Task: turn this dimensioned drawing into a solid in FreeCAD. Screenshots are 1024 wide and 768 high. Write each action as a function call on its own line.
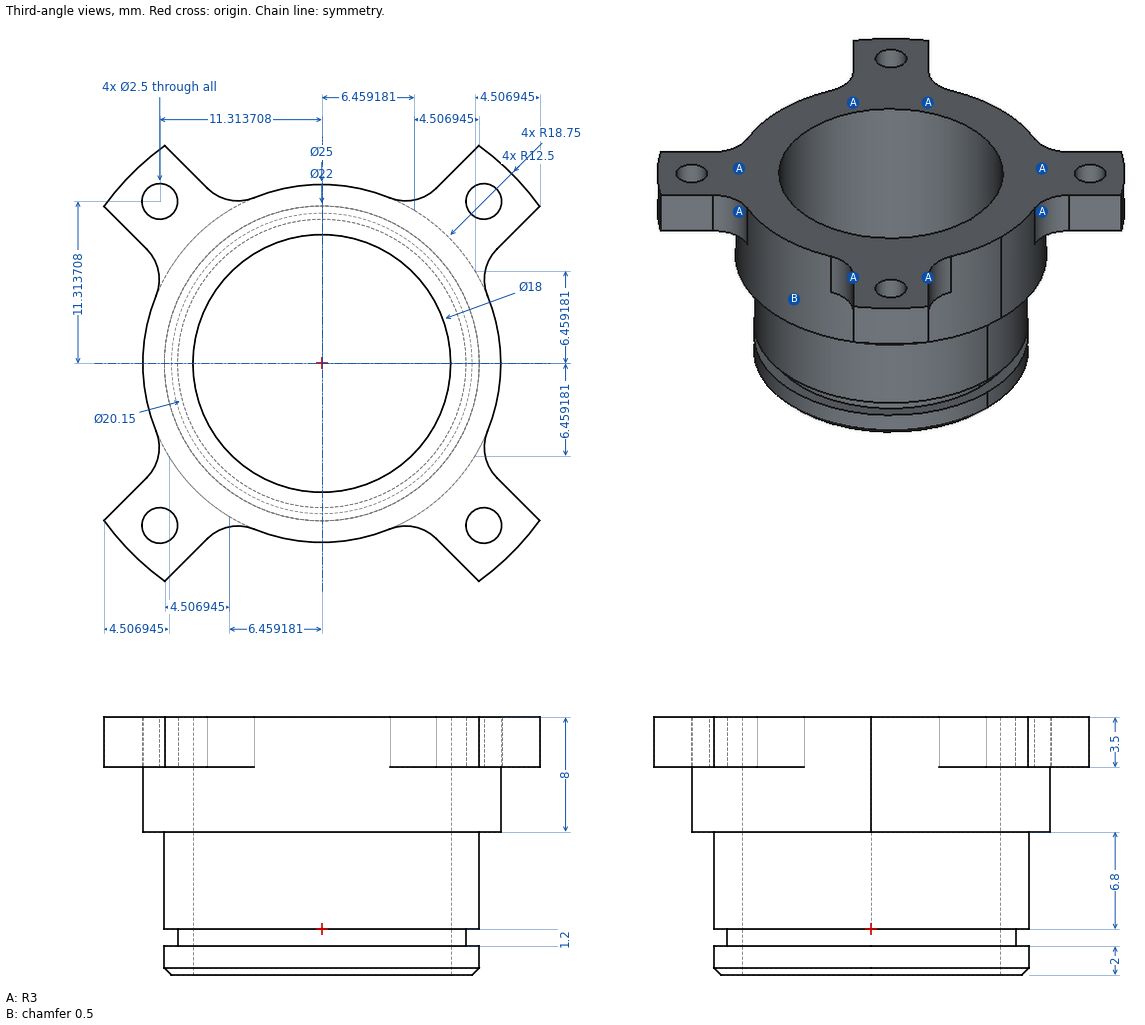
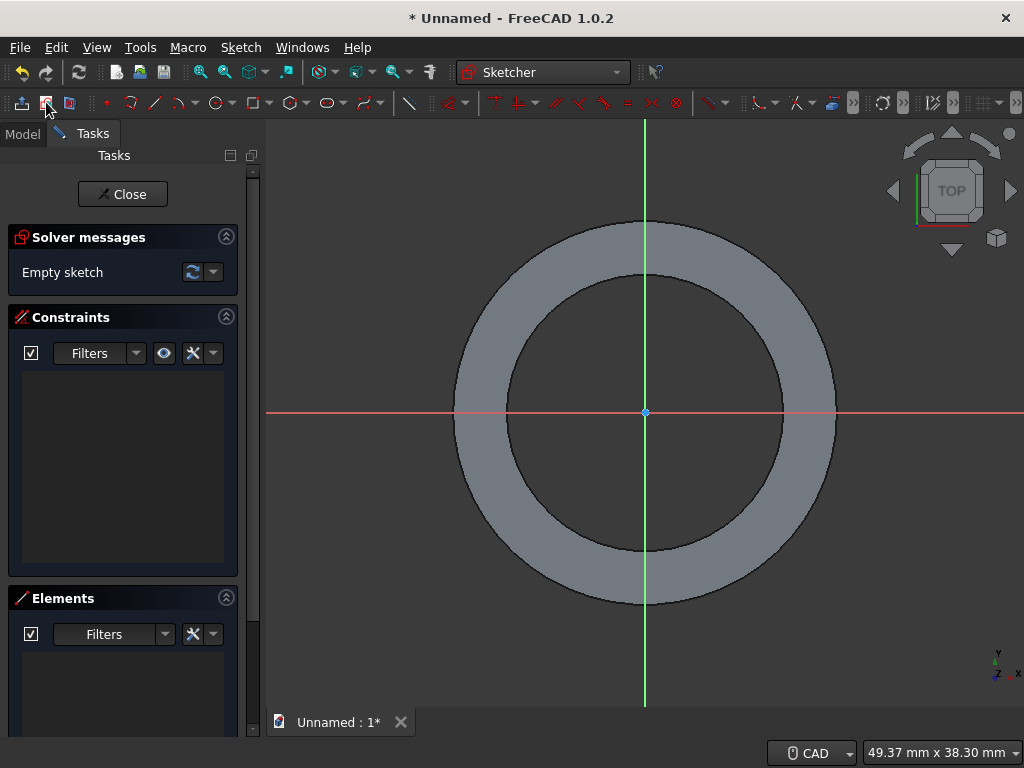
scroll(294, 413, down, 1)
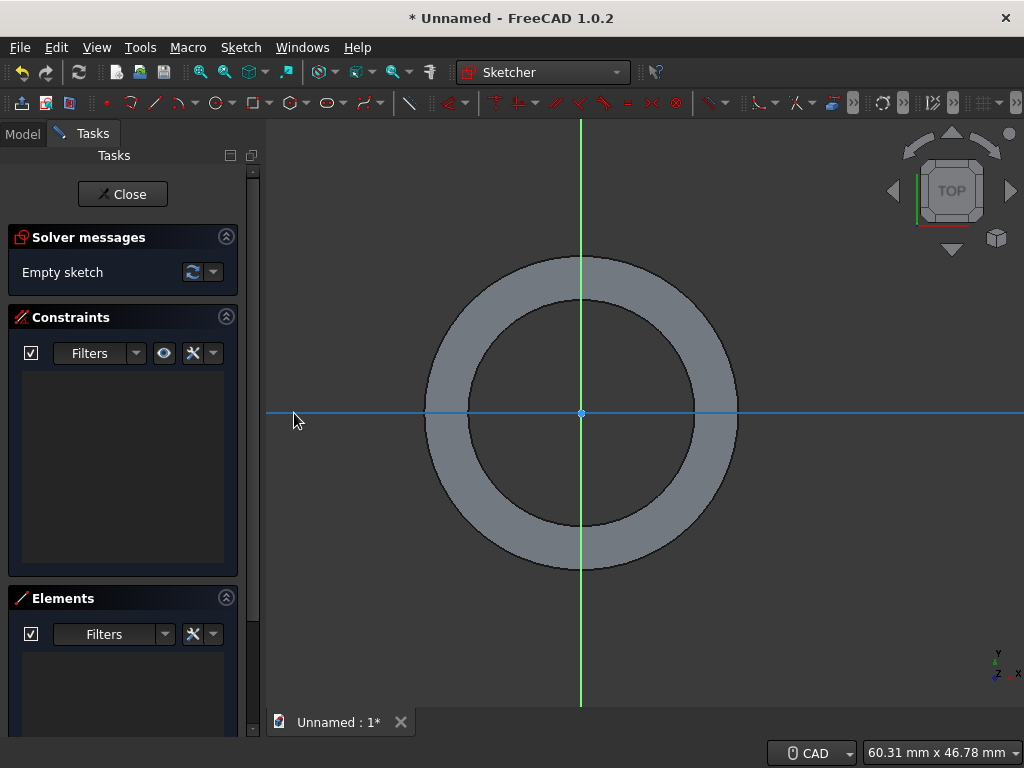
click(216, 104)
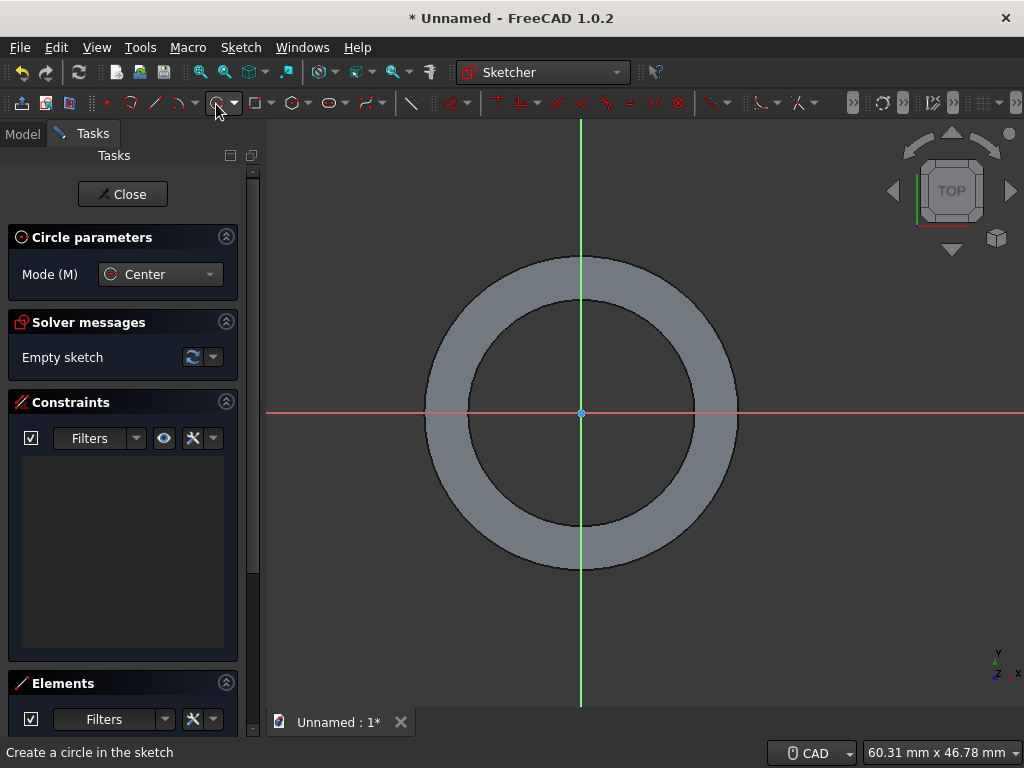
click(581, 413)
click(692, 302)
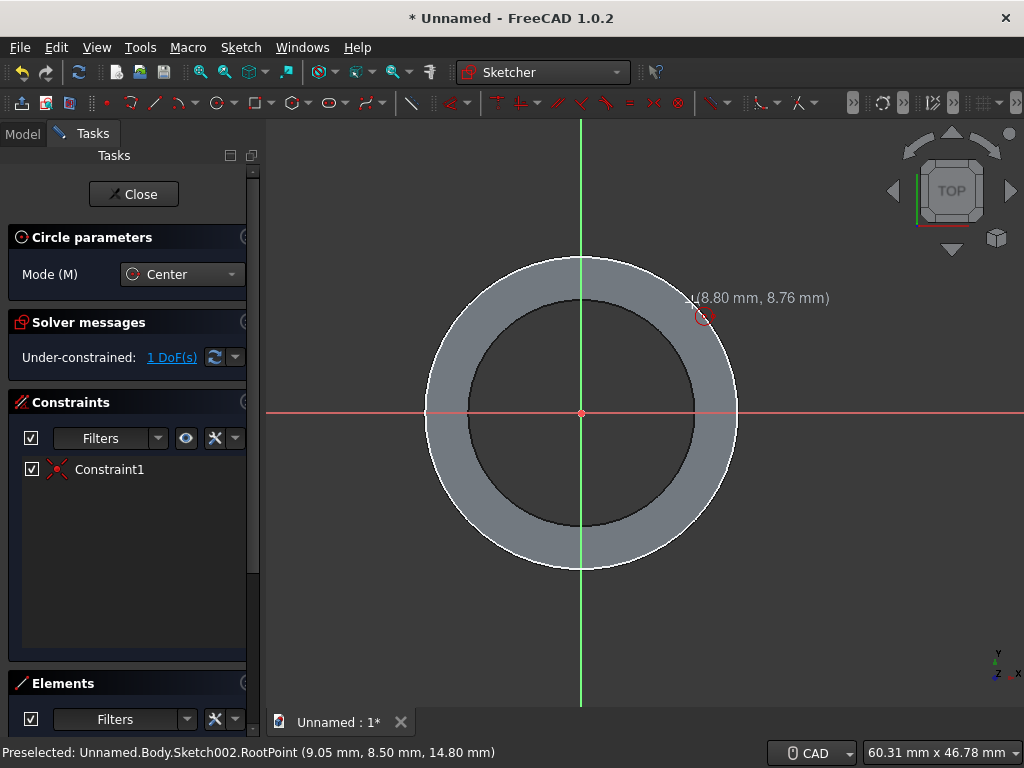
click(581, 413)
click(661, 333)
key(Escape)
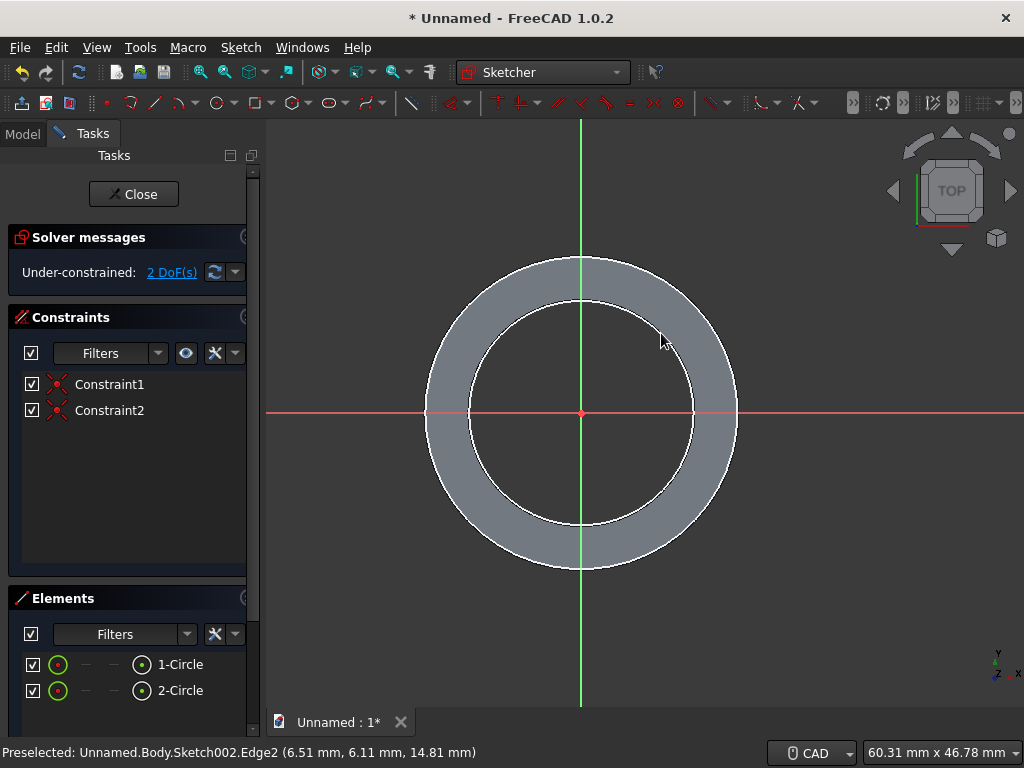
click(450, 104)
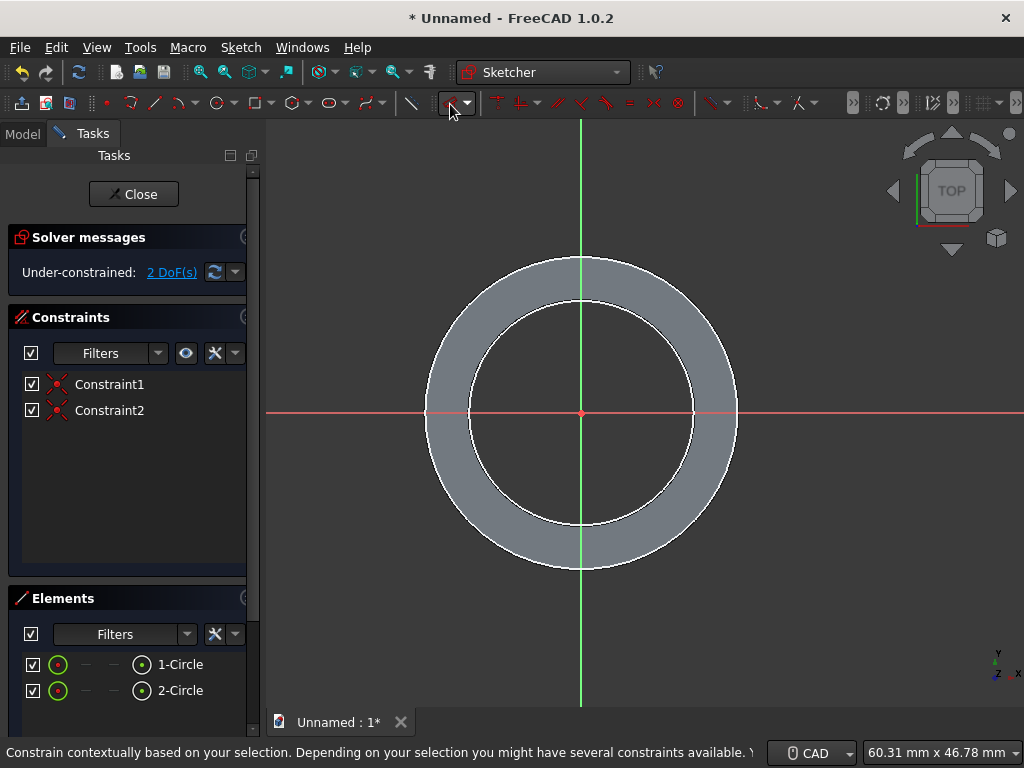
click(691, 302)
click(713, 279)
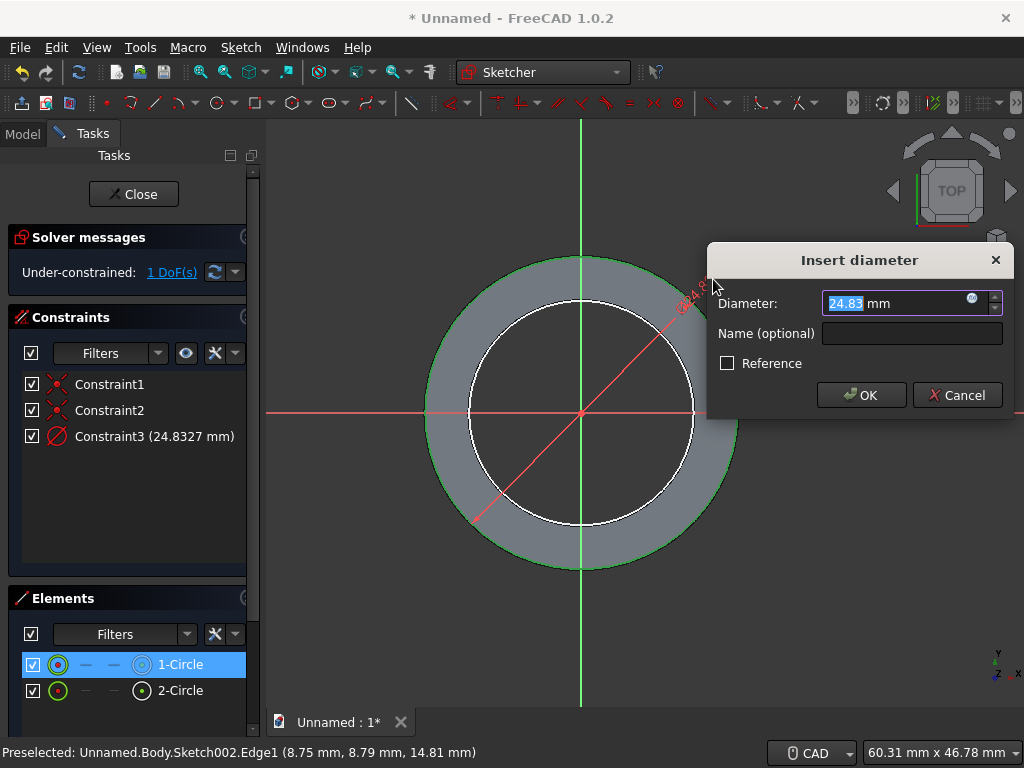
text(25)
key(Return)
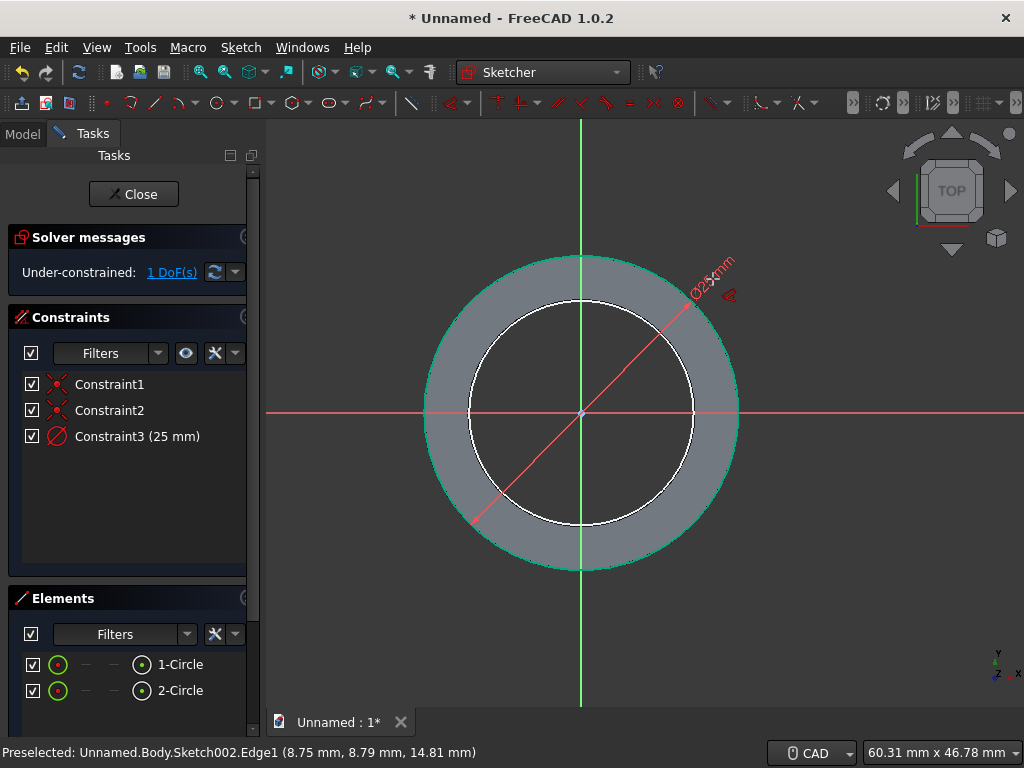
click(660, 333)
click(765, 357)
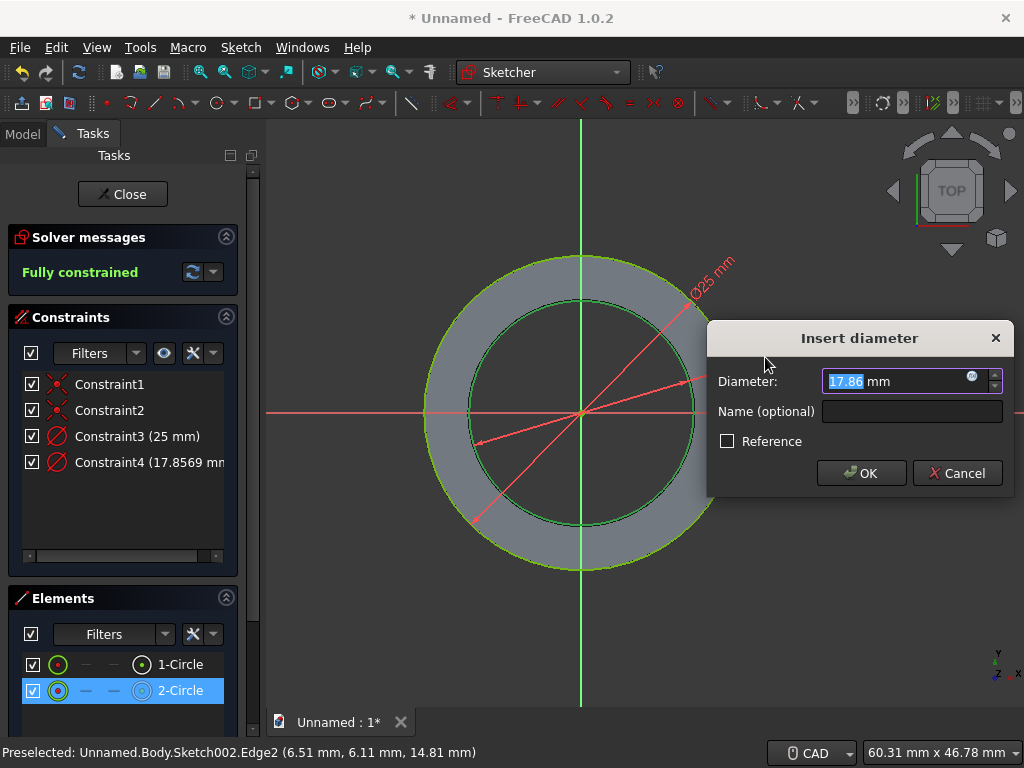
text(18)
key(Return)
key(Escape)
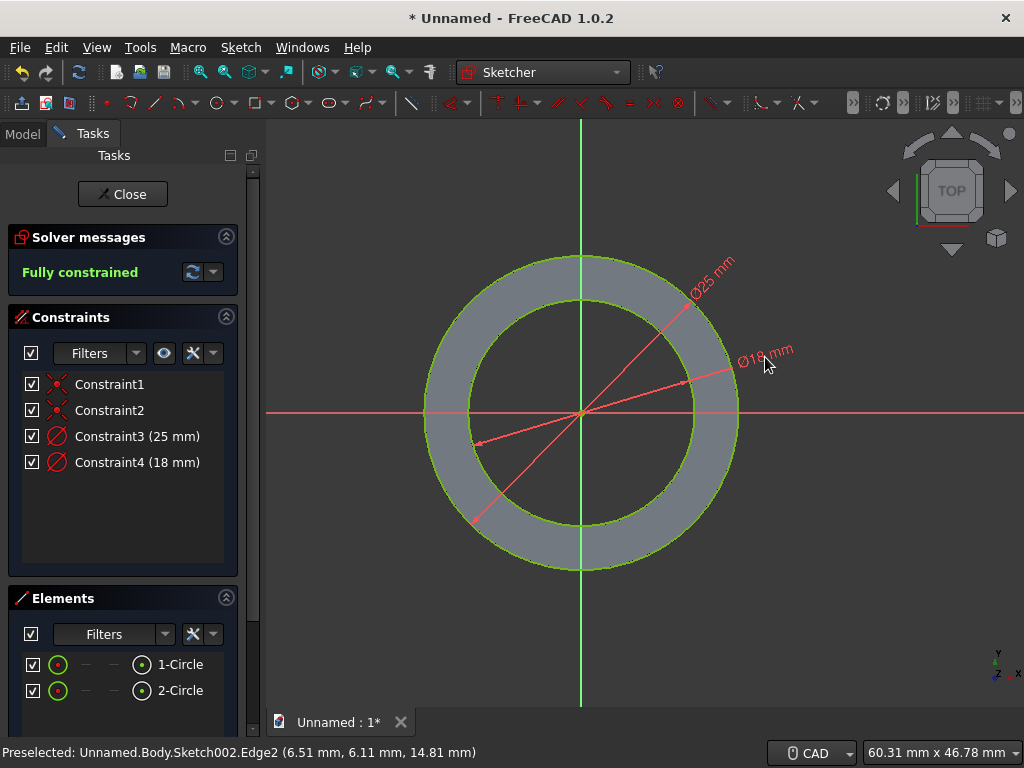
click(123, 194)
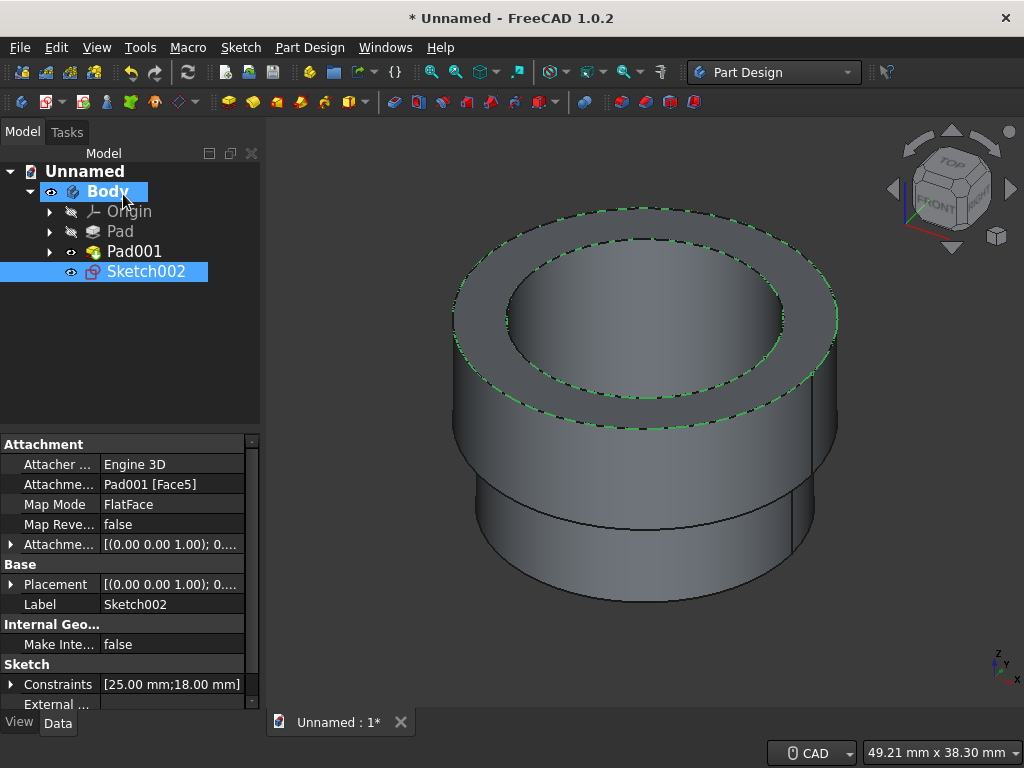
click(230, 102)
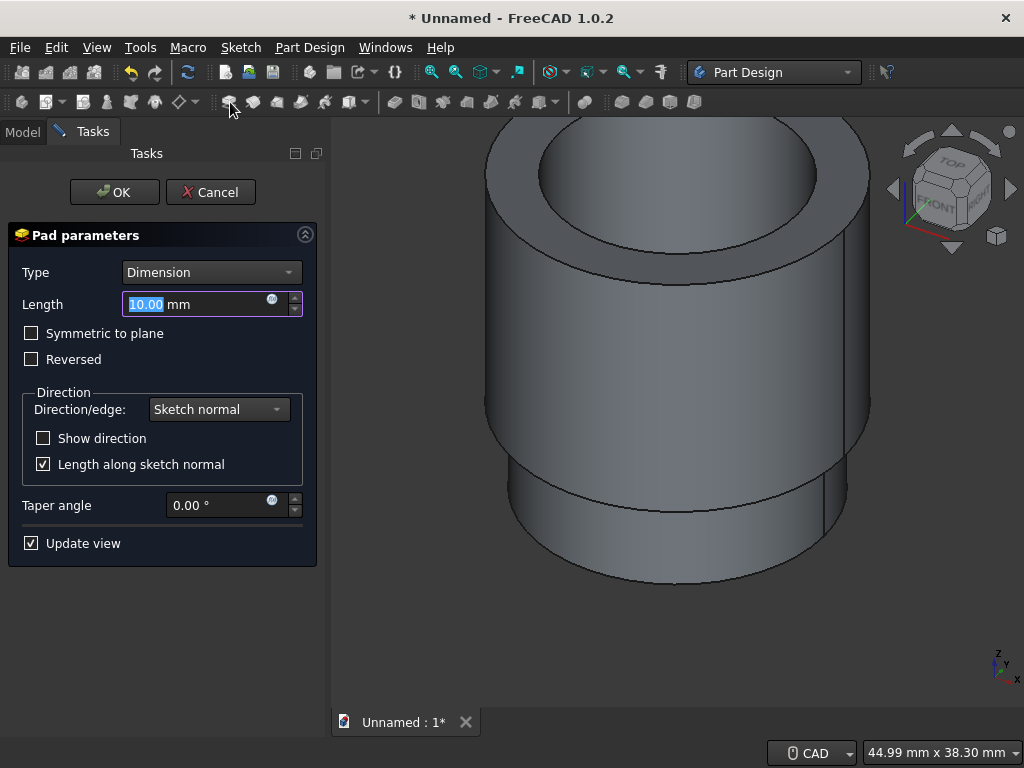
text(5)
key(Tab)